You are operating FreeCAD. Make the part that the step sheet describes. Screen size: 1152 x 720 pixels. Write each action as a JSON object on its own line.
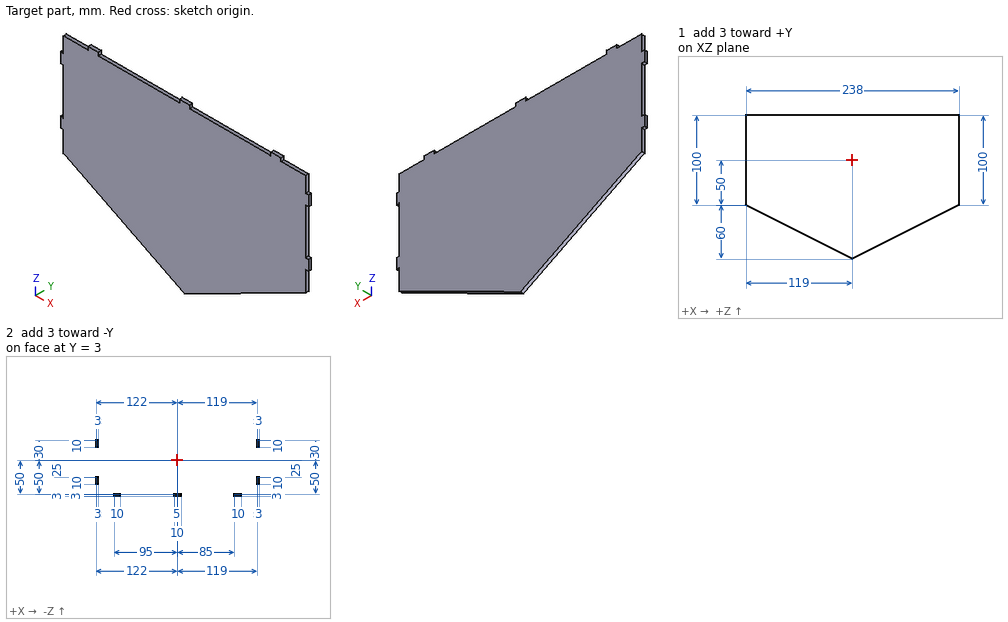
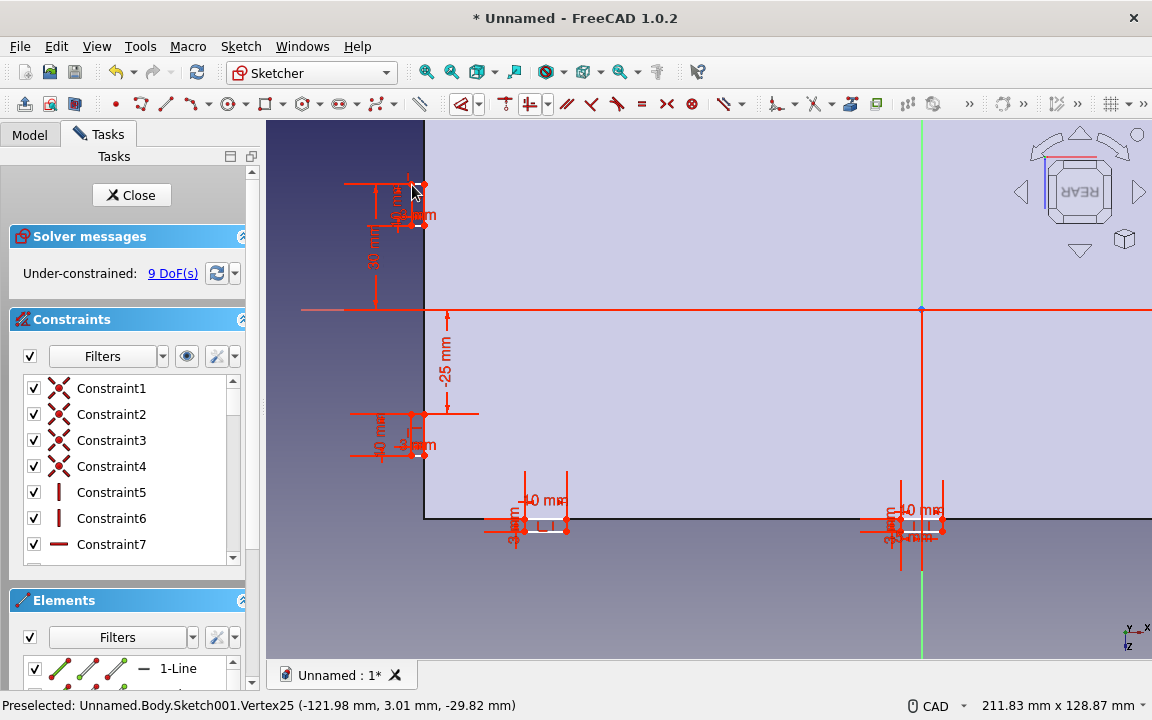
{"action": "left_click", "coordinate": [525, 519]}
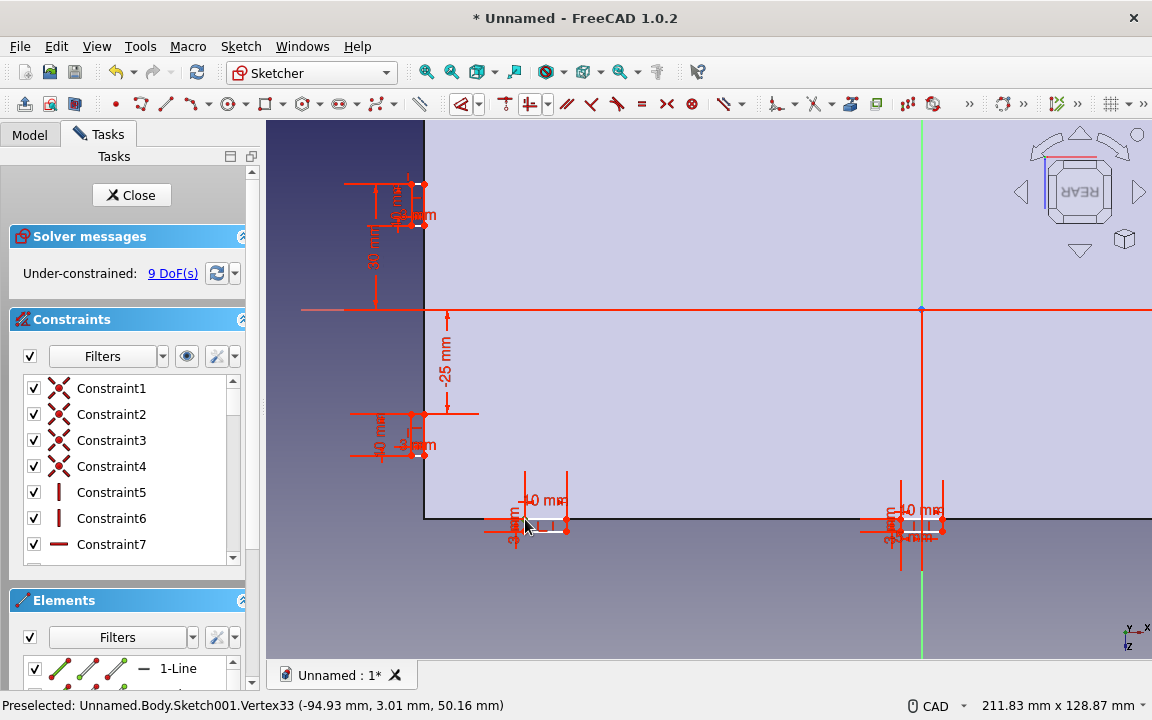
{"action": "key", "text": "l"}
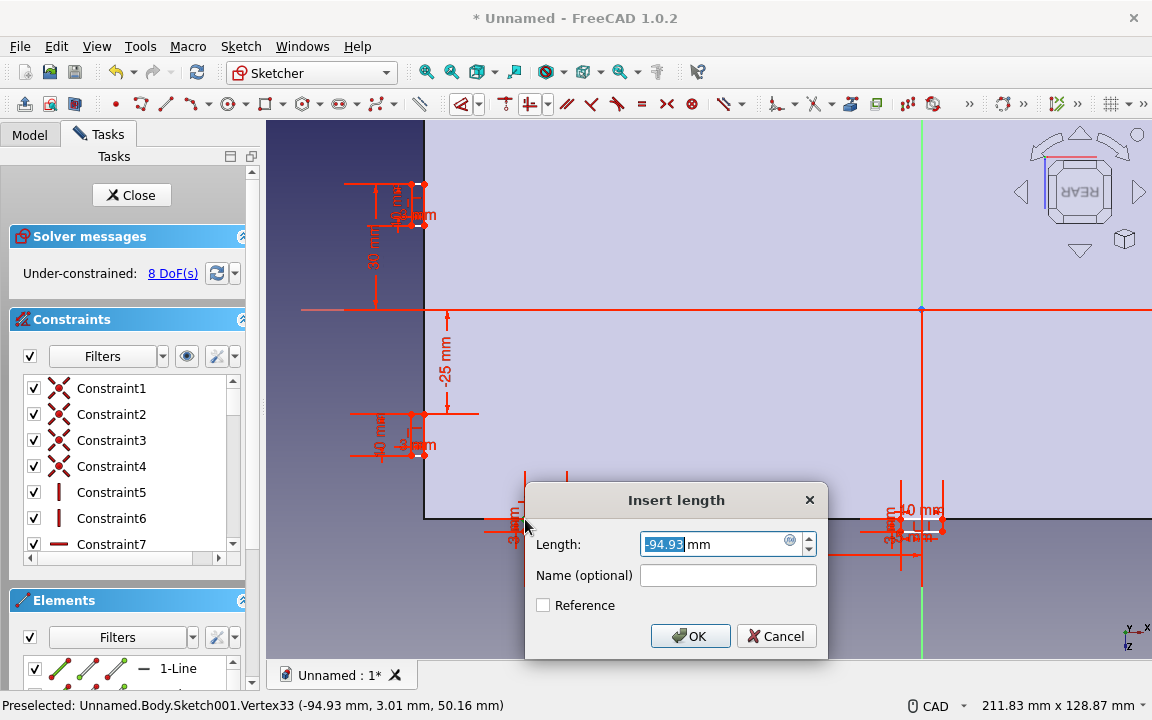
{"action": "type", "text": "-95"}
{"action": "key", "text": "Return"}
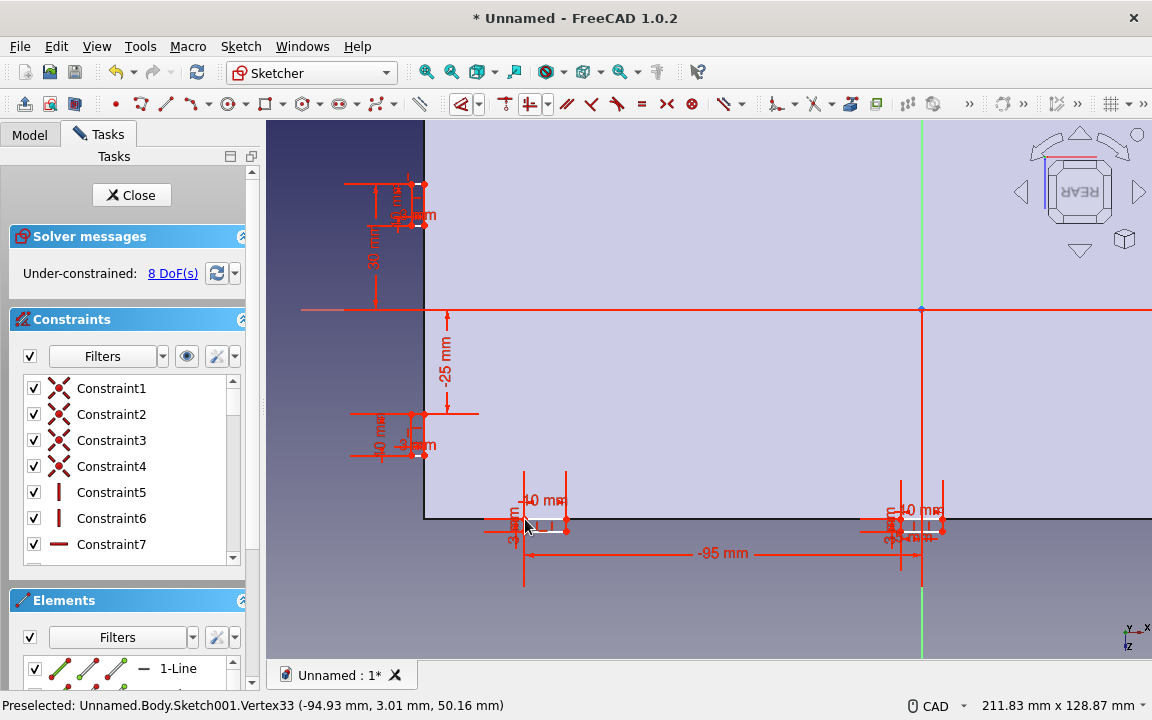
{"action": "left_click", "coordinate": [525, 519]}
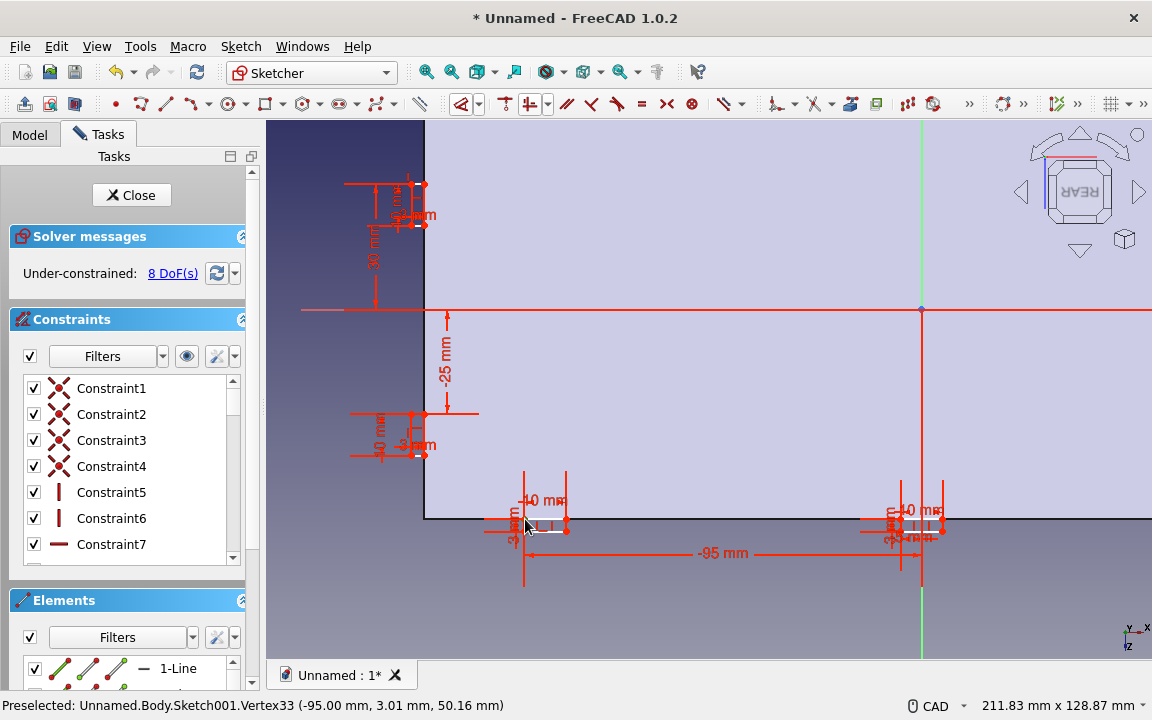
{"action": "key", "text": "i"}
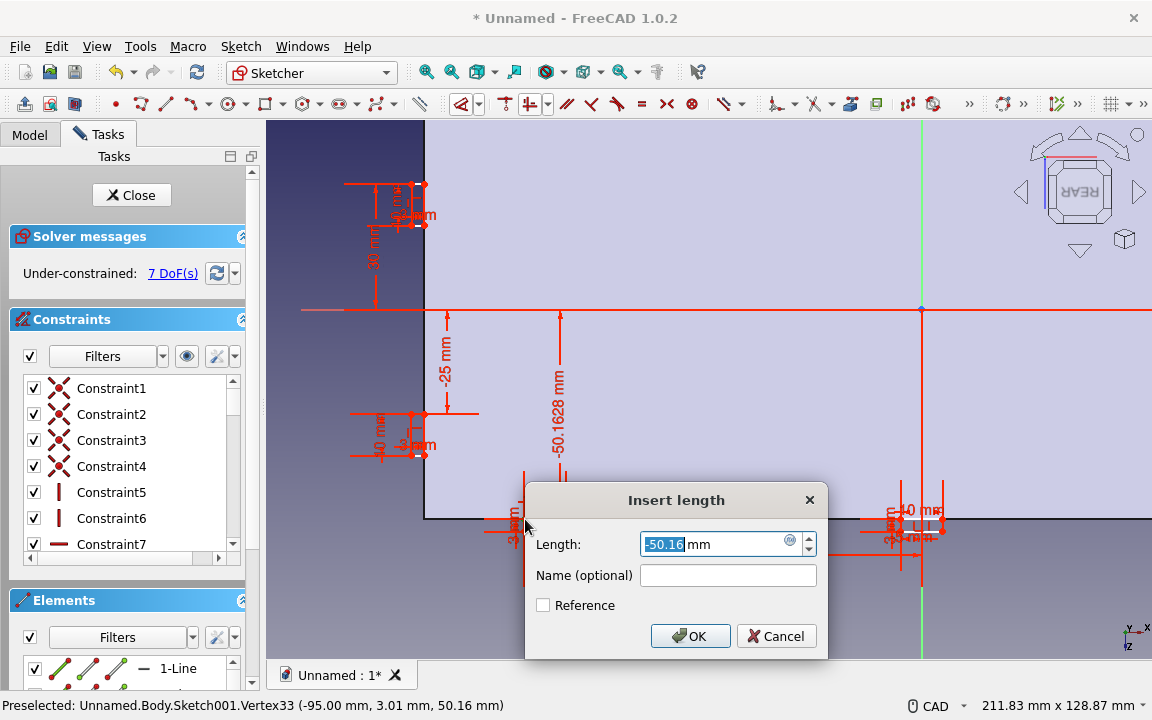
{"action": "type", "text": "-50"}
{"action": "key", "text": "Return"}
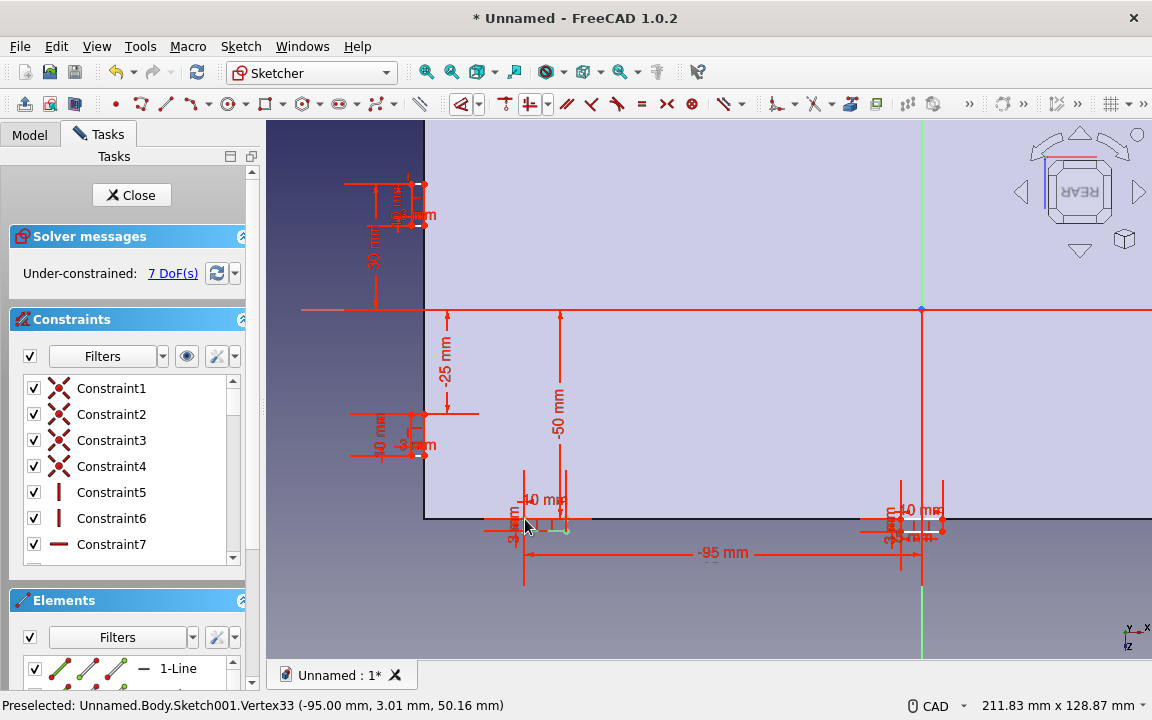
{"action": "scroll", "coordinate": [411, 416], "scroll_direction": "down", "scroll_amount": 4}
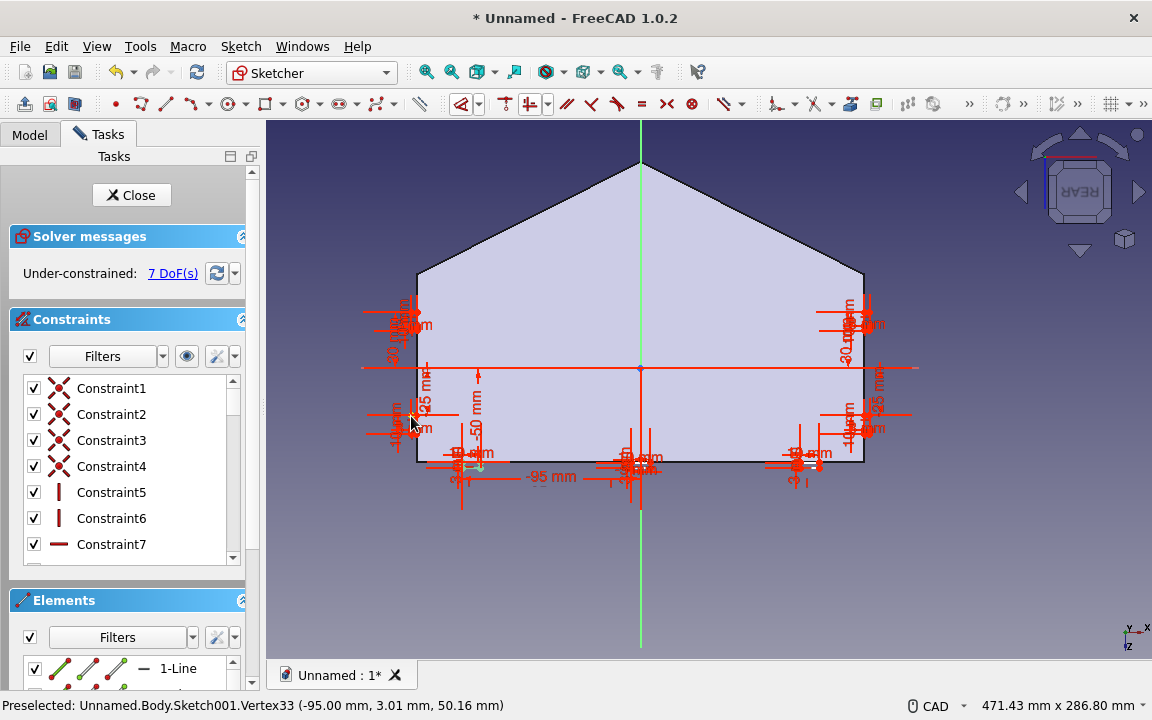
{"action": "scroll", "coordinate": [800, 463], "scroll_direction": "up", "scroll_amount": 4}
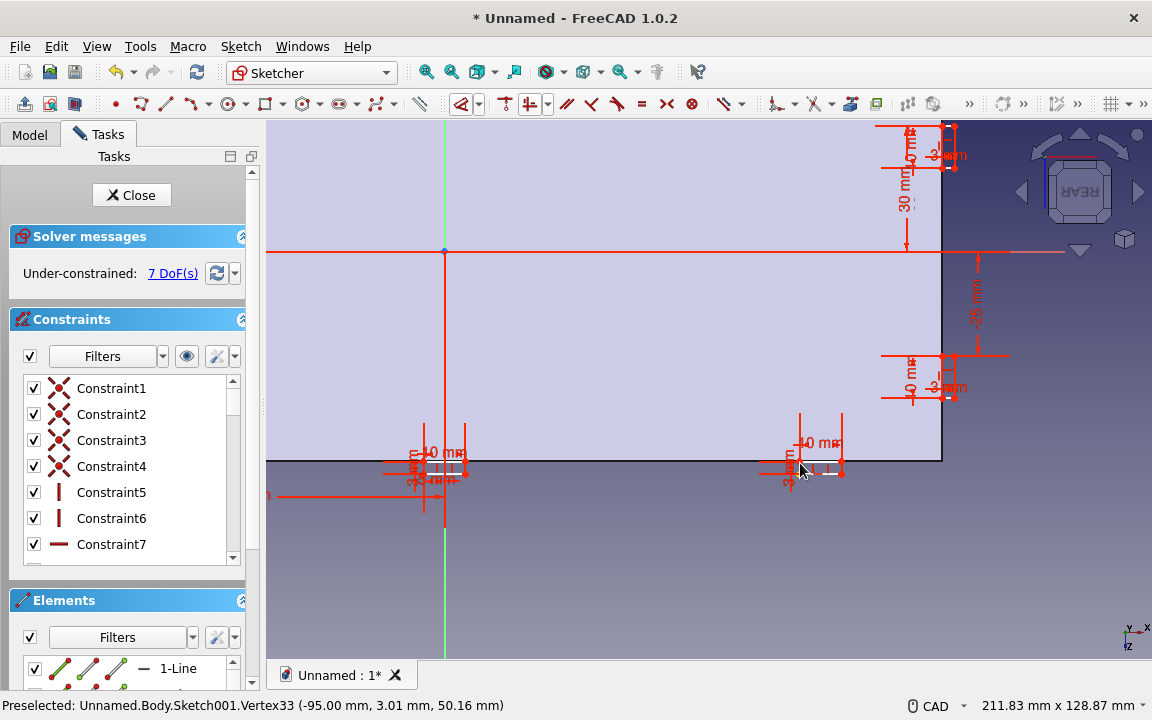
{"action": "left_click", "coordinate": [800, 462]}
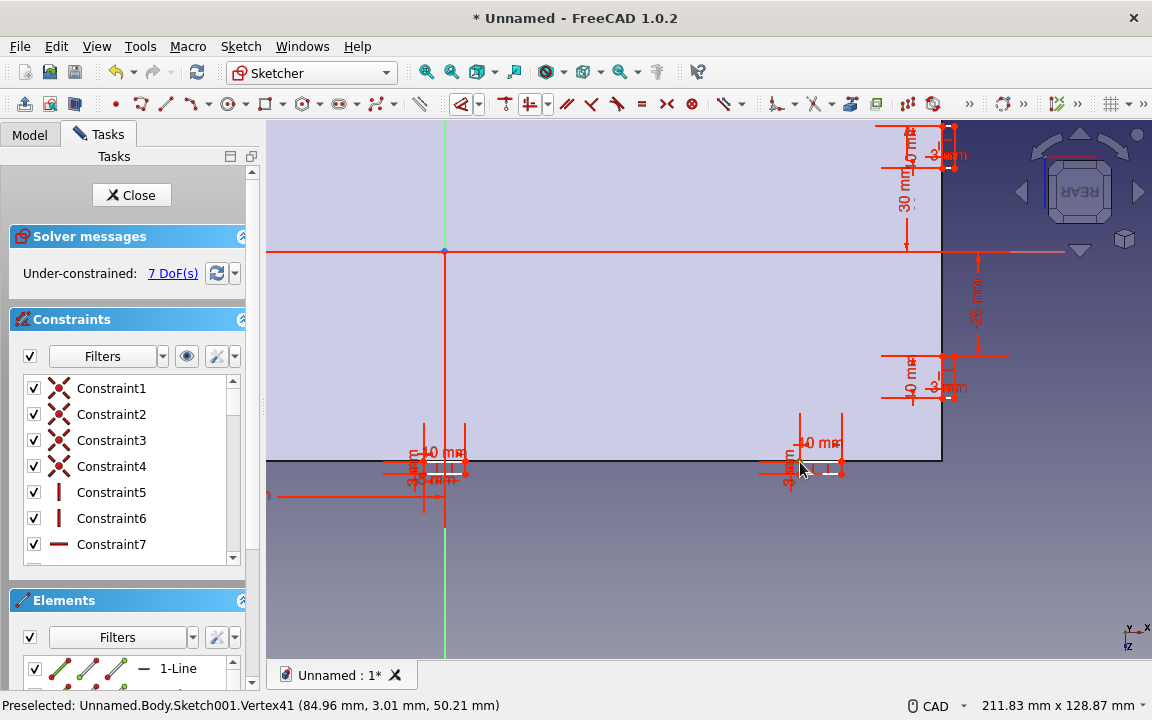
{"action": "key", "text": "l"}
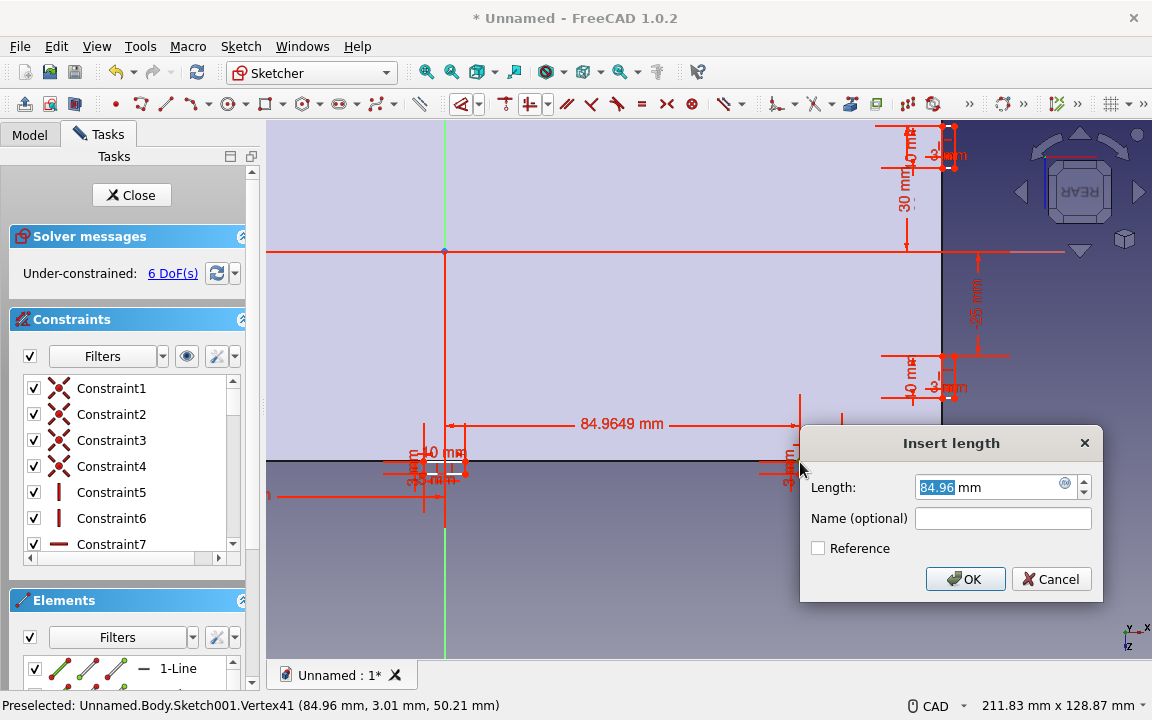
{"action": "type", "text": "85"}
{"action": "key", "text": "Return"}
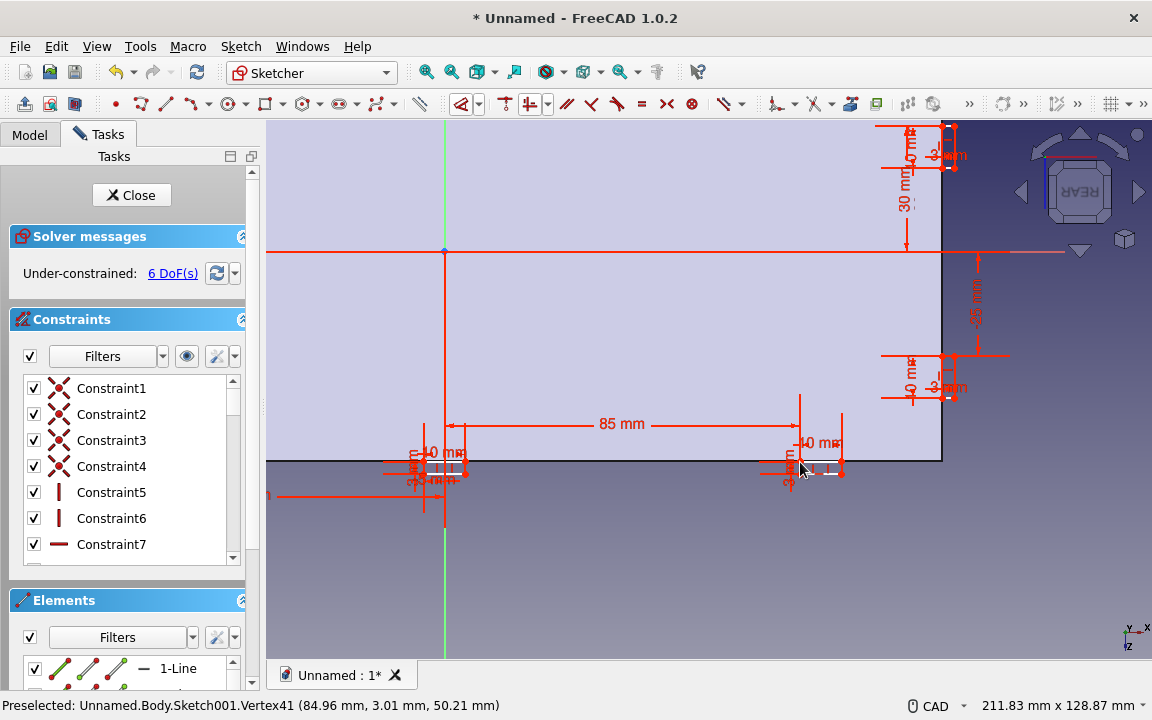
{"action": "left_click", "coordinate": [800, 462]}